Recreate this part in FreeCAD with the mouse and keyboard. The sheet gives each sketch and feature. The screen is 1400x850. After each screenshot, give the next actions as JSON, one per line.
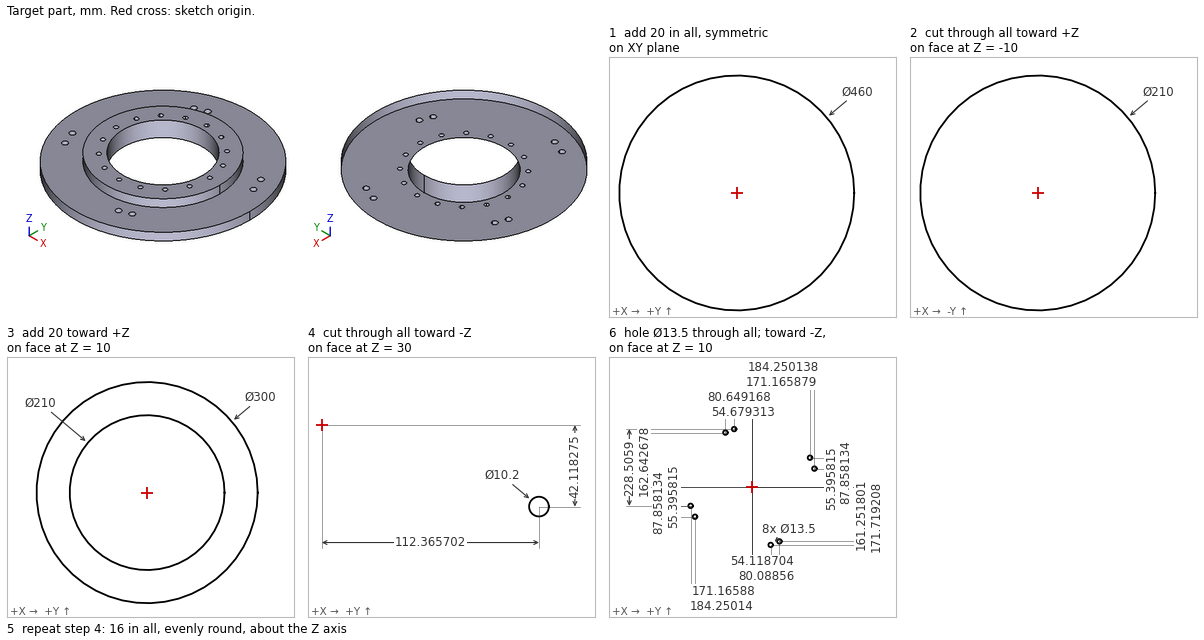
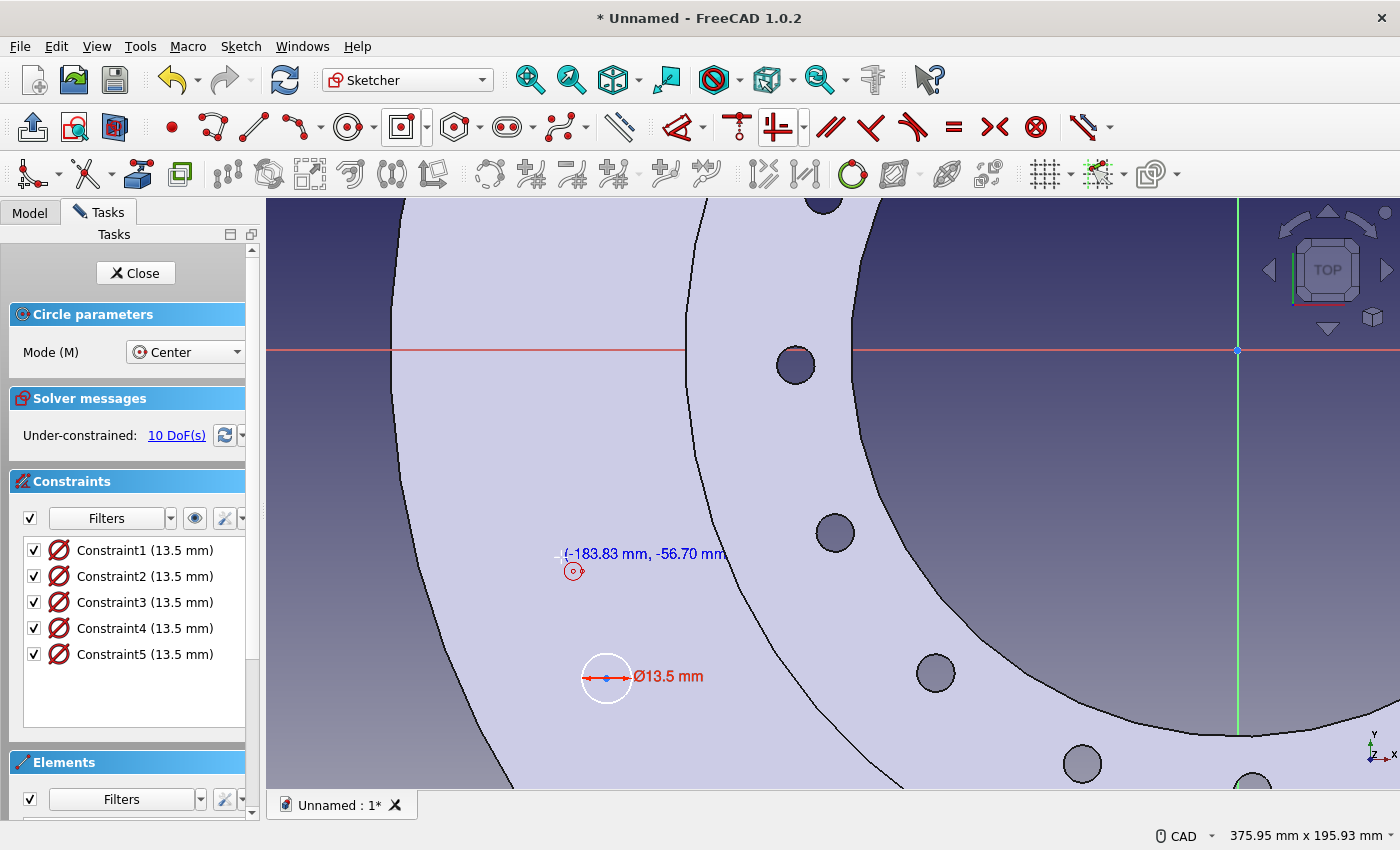
{"action": "scroll", "coordinate": [561, 556], "scroll_direction": "down", "scroll_amount": 6}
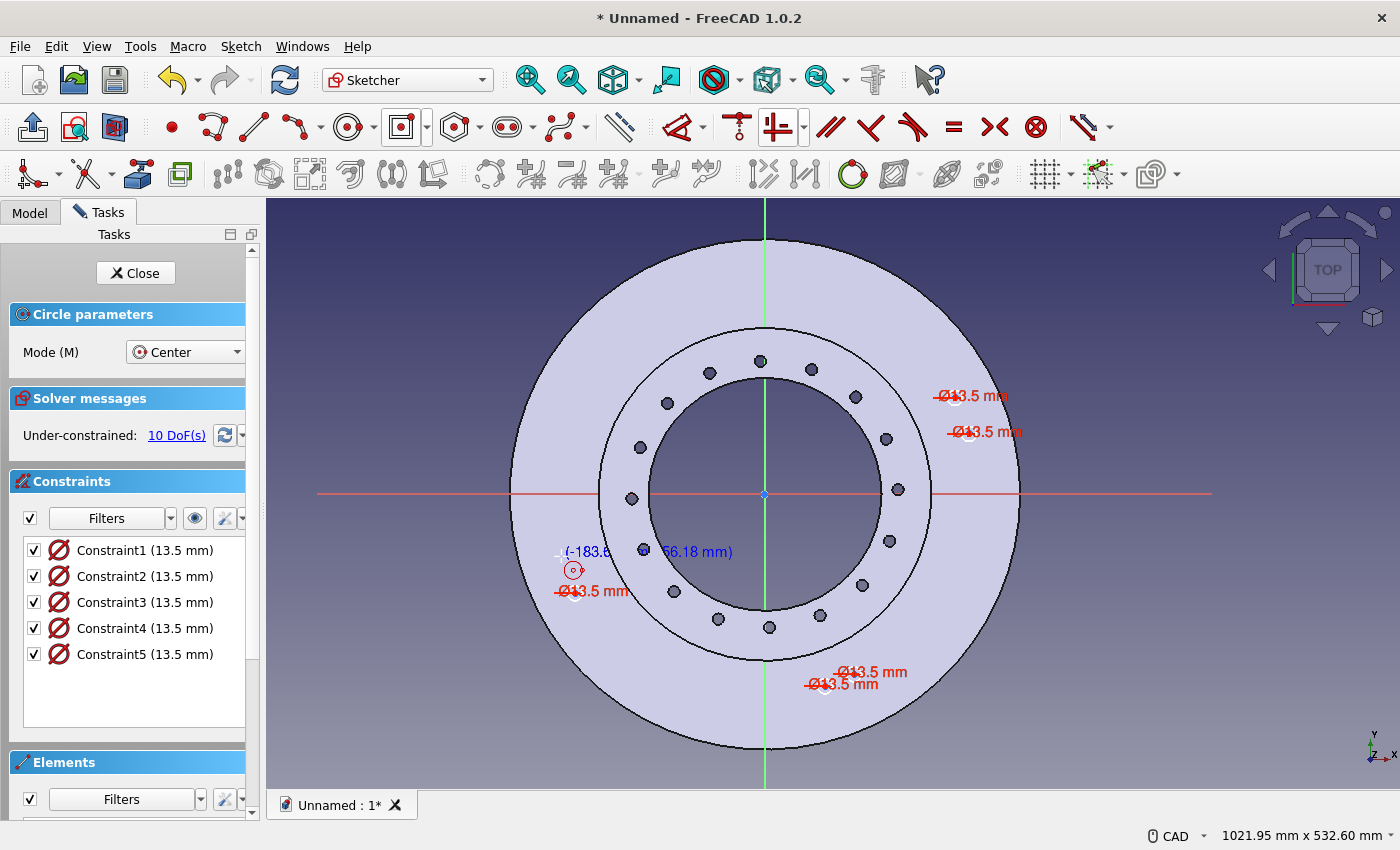
{"action": "left_click", "coordinate": [561, 556]}
{"action": "mouse_move", "coordinate": [566, 551]}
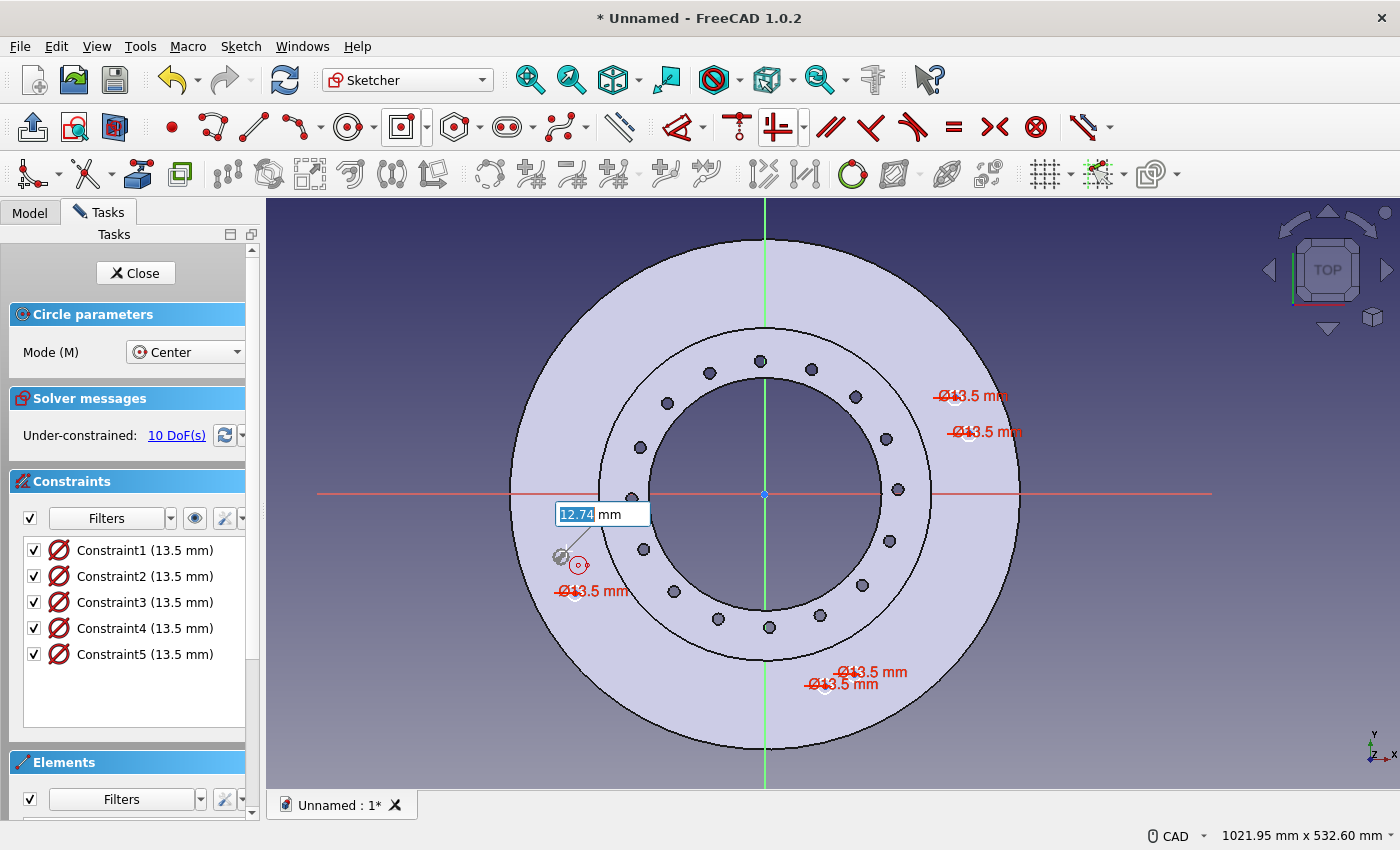
{"action": "type", "text": "13.5"}
{"action": "key", "text": "Return"}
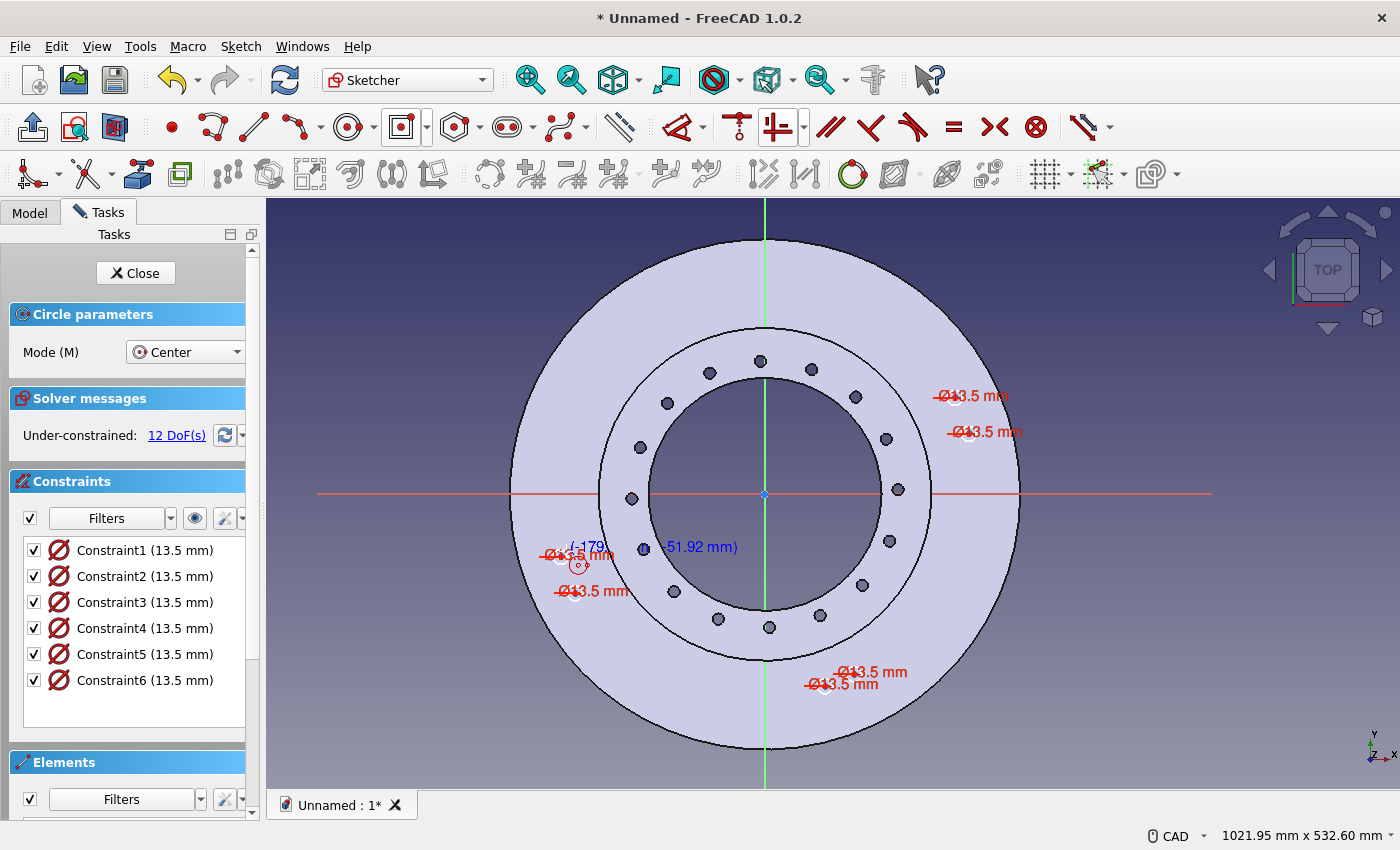
{"action": "scroll", "coordinate": [675, 314], "scroll_direction": "up", "scroll_amount": 6}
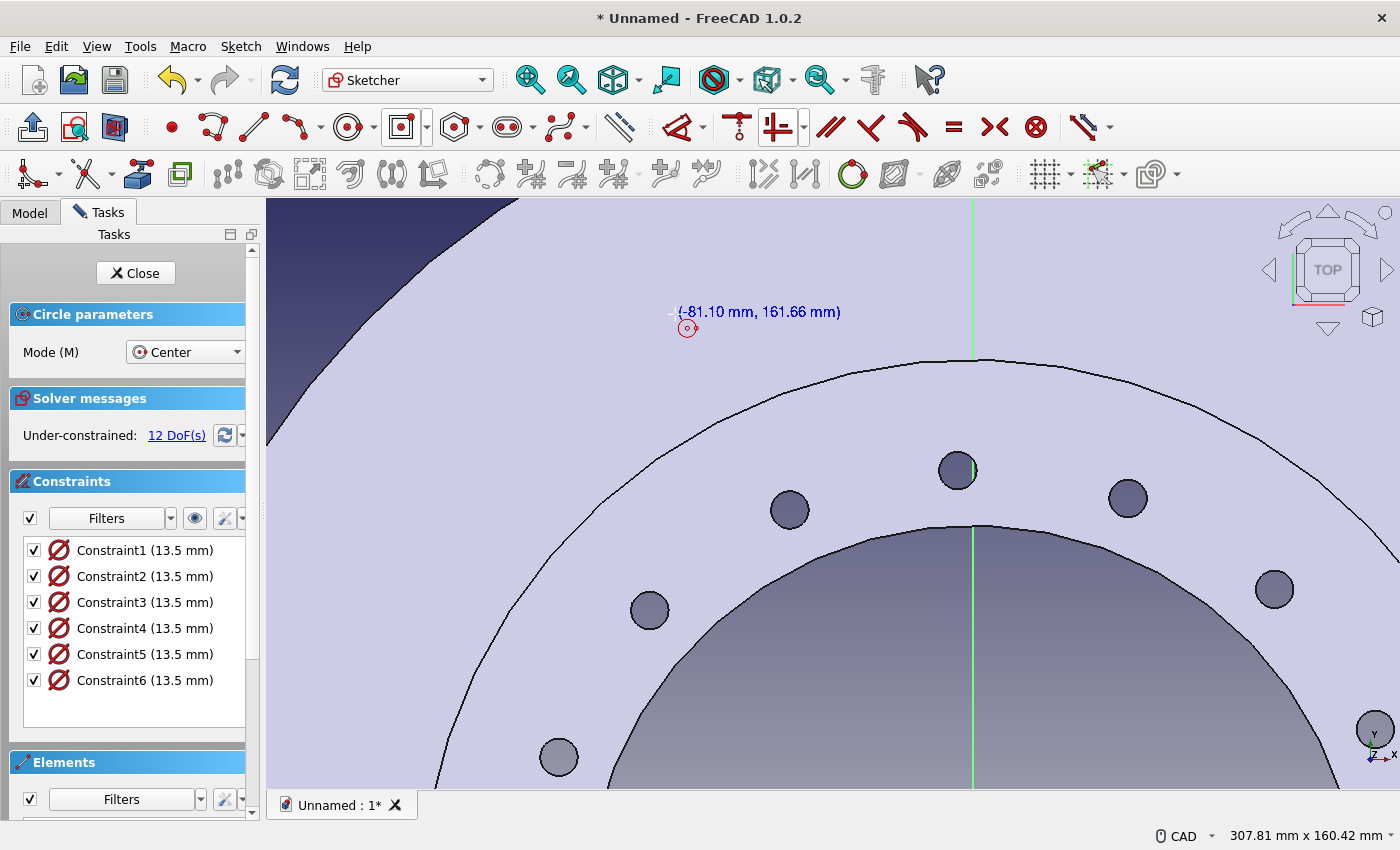
{"action": "scroll", "coordinate": [675, 314], "scroll_direction": "down", "scroll_amount": 6}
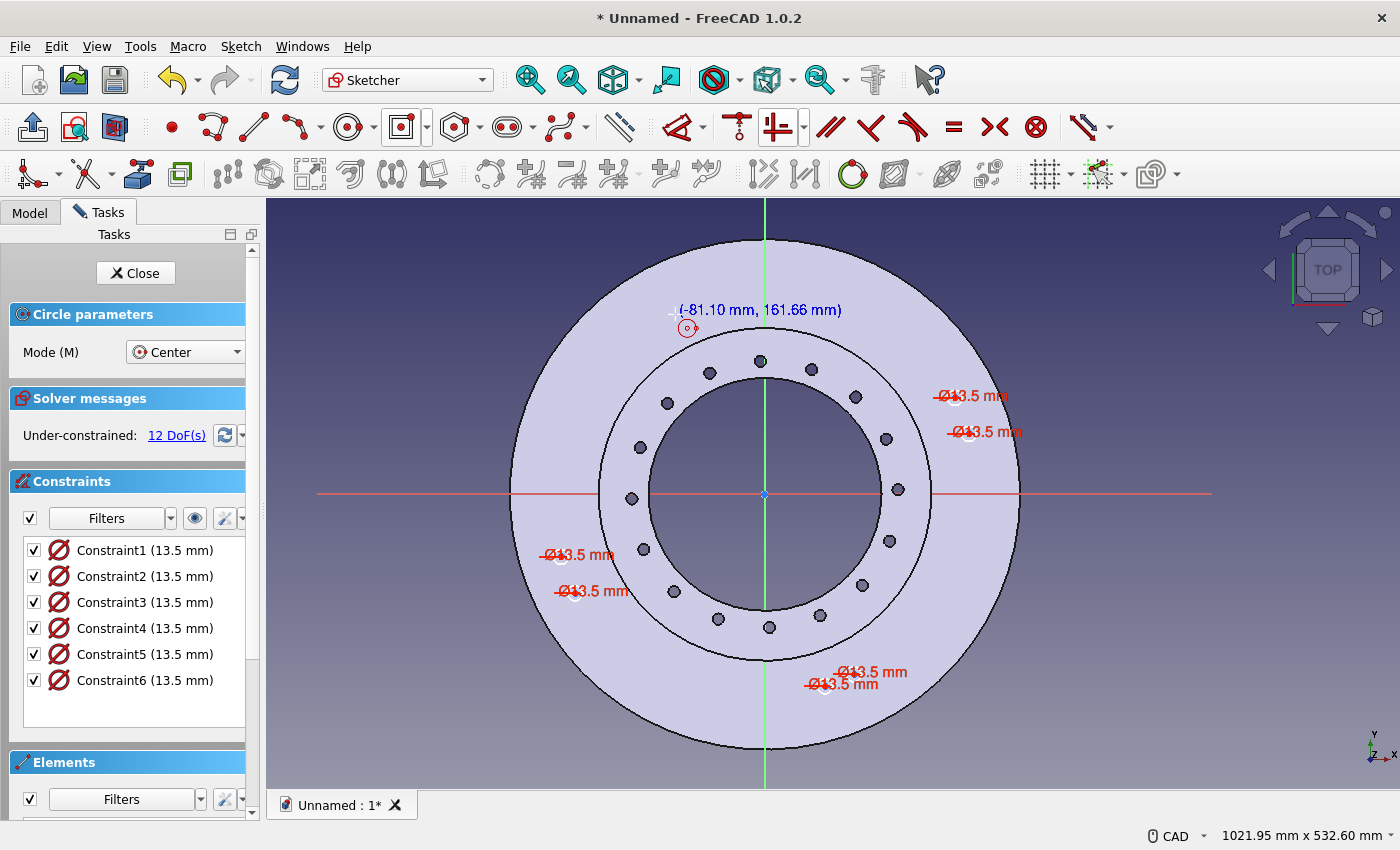
{"action": "left_click", "coordinate": [675, 314]}
{"action": "mouse_move", "coordinate": [681, 309]}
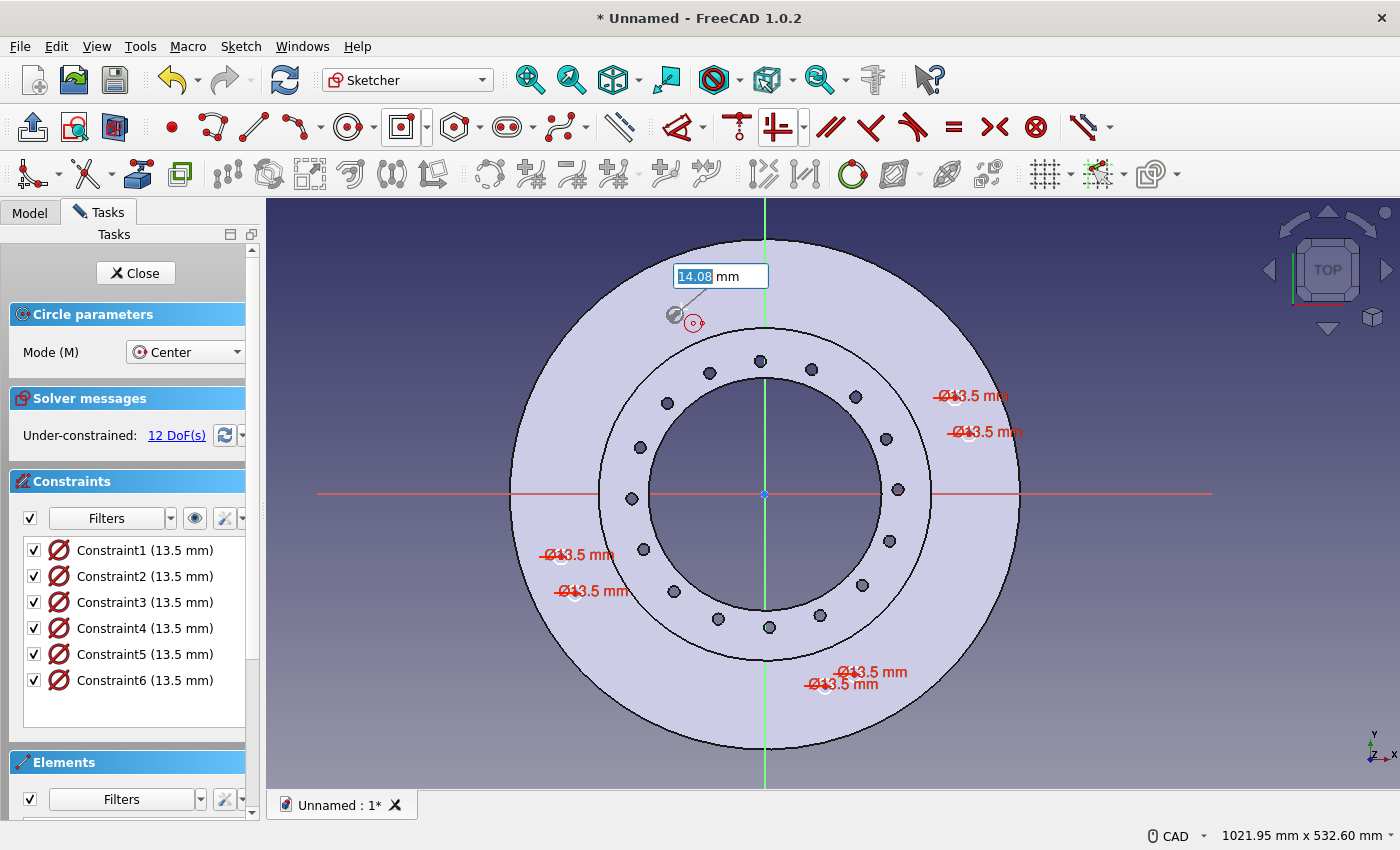
{"action": "type", "text": "13.5"}
{"action": "key", "text": "Return"}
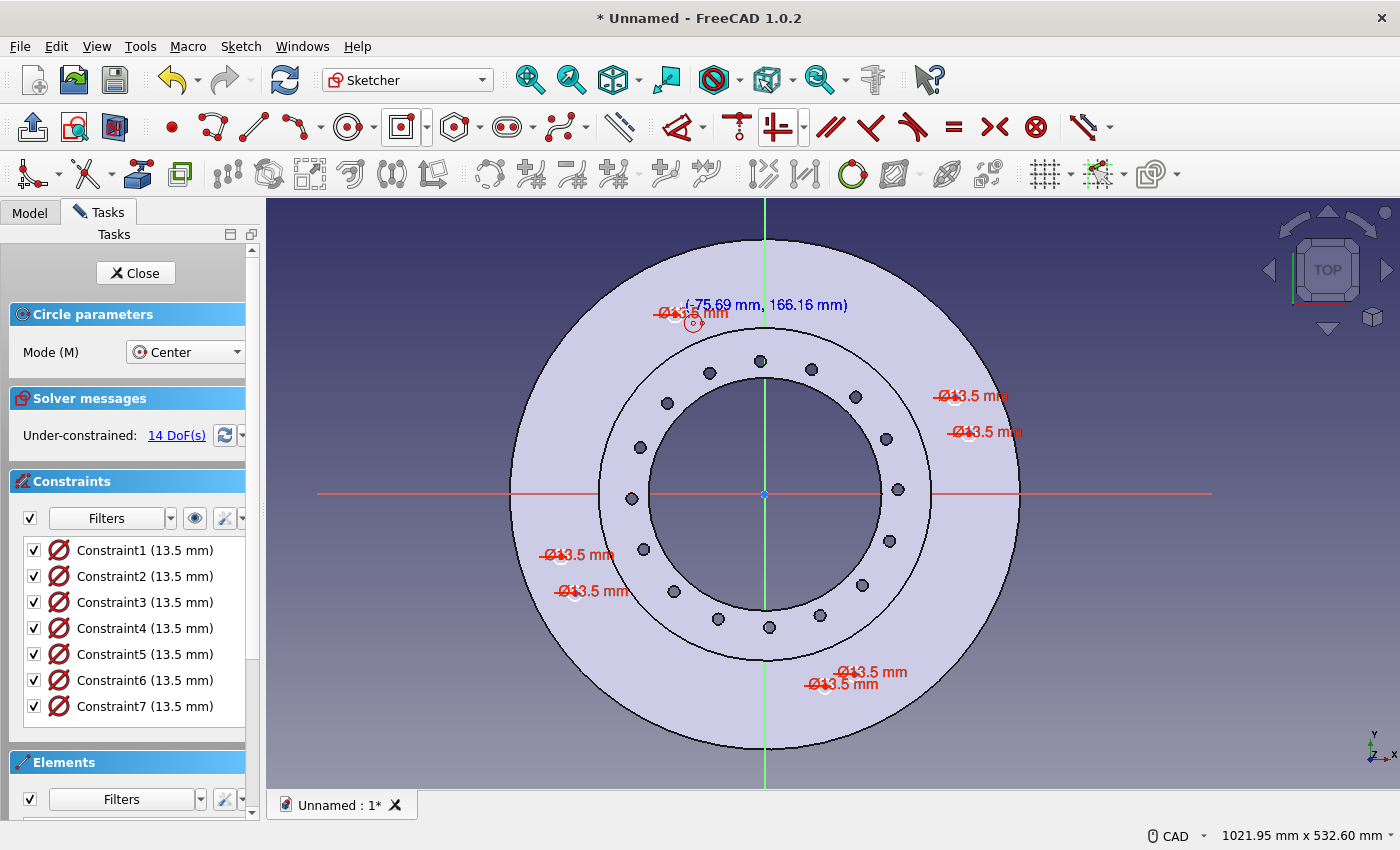
{"action": "scroll", "coordinate": [704, 302], "scroll_direction": "up", "scroll_amount": 6}